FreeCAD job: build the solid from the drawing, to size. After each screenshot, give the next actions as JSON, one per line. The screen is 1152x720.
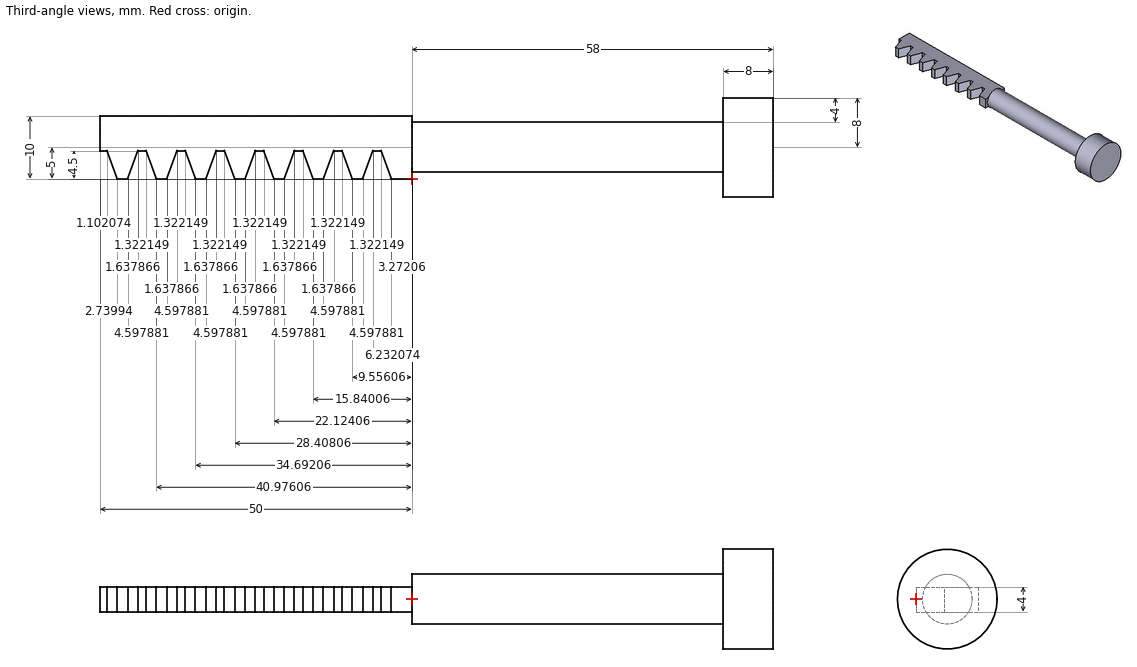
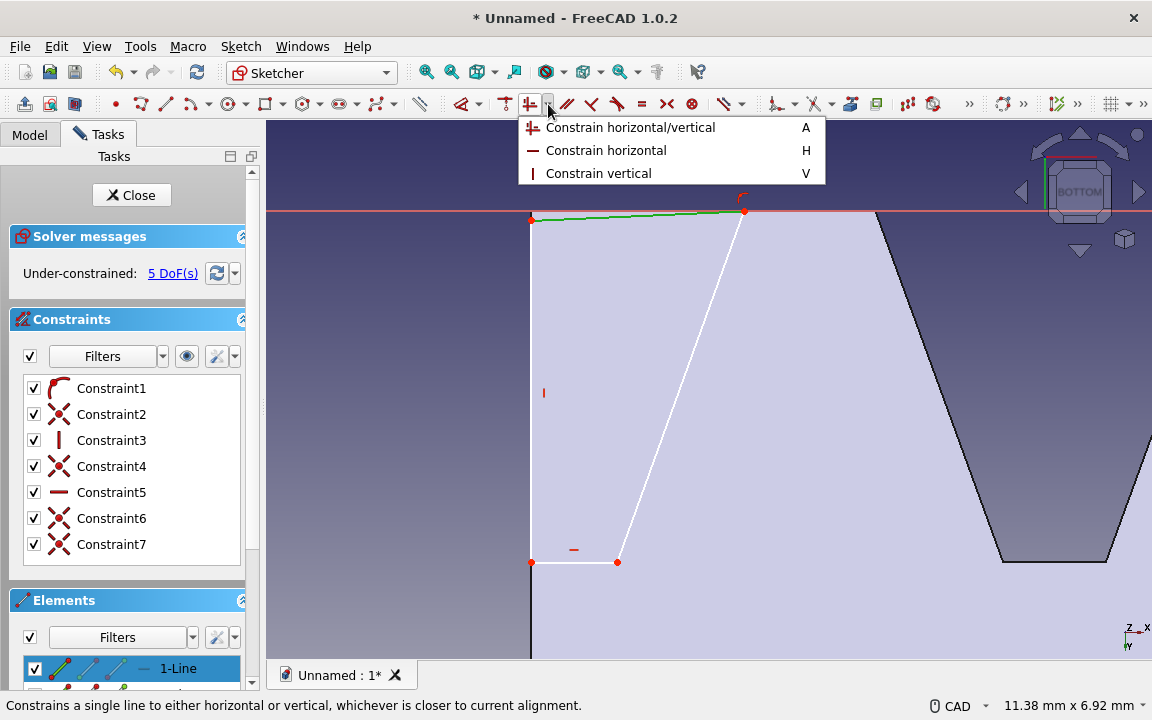
{"action": "left_click", "coordinate": [672, 150]}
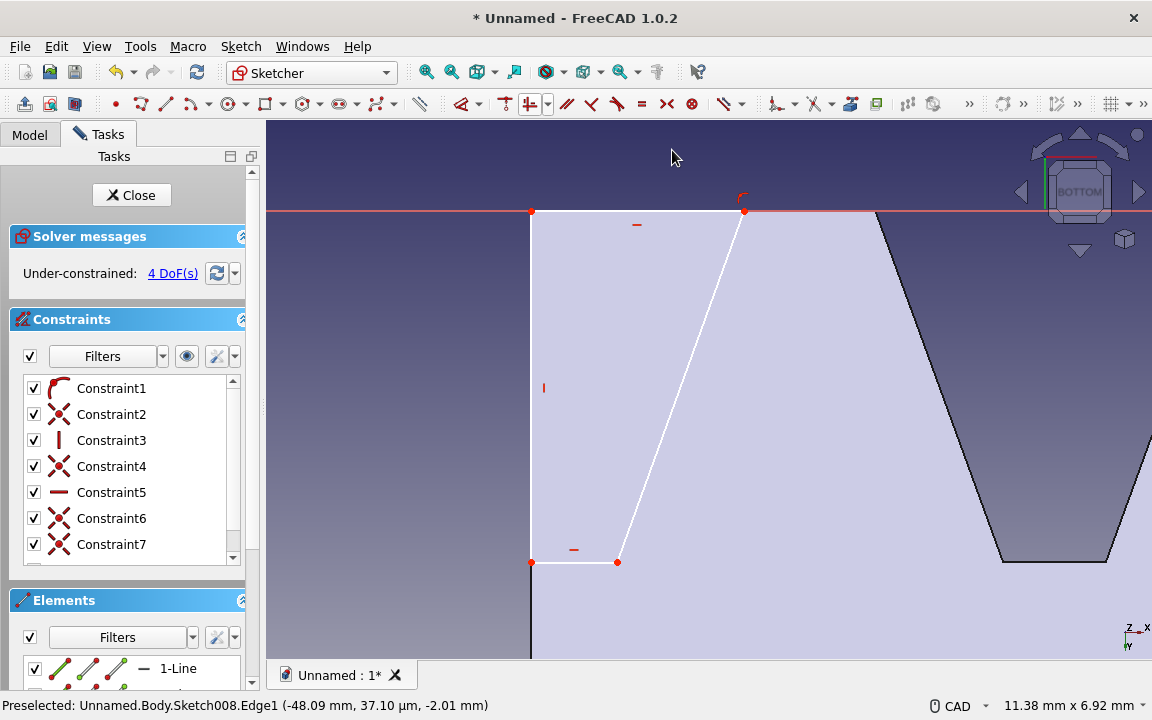
{"action": "left_click", "coordinate": [460, 104]}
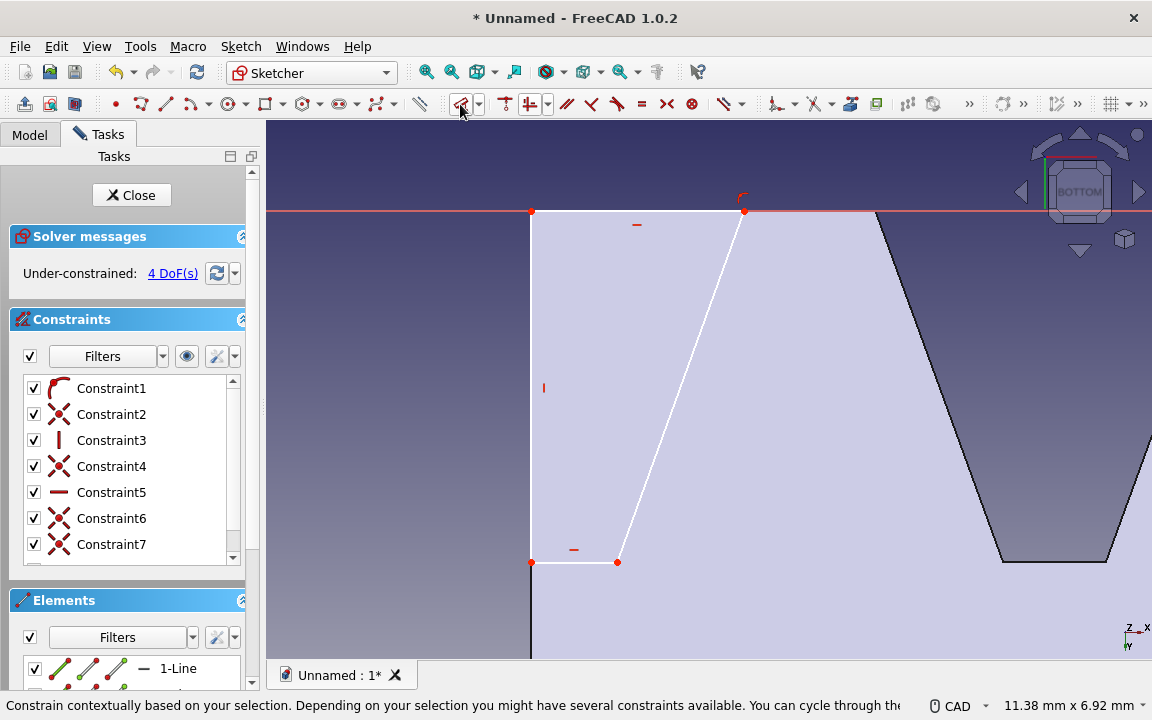
{"action": "left_click", "coordinate": [531, 317]}
{"action": "left_click", "coordinate": [497, 387]}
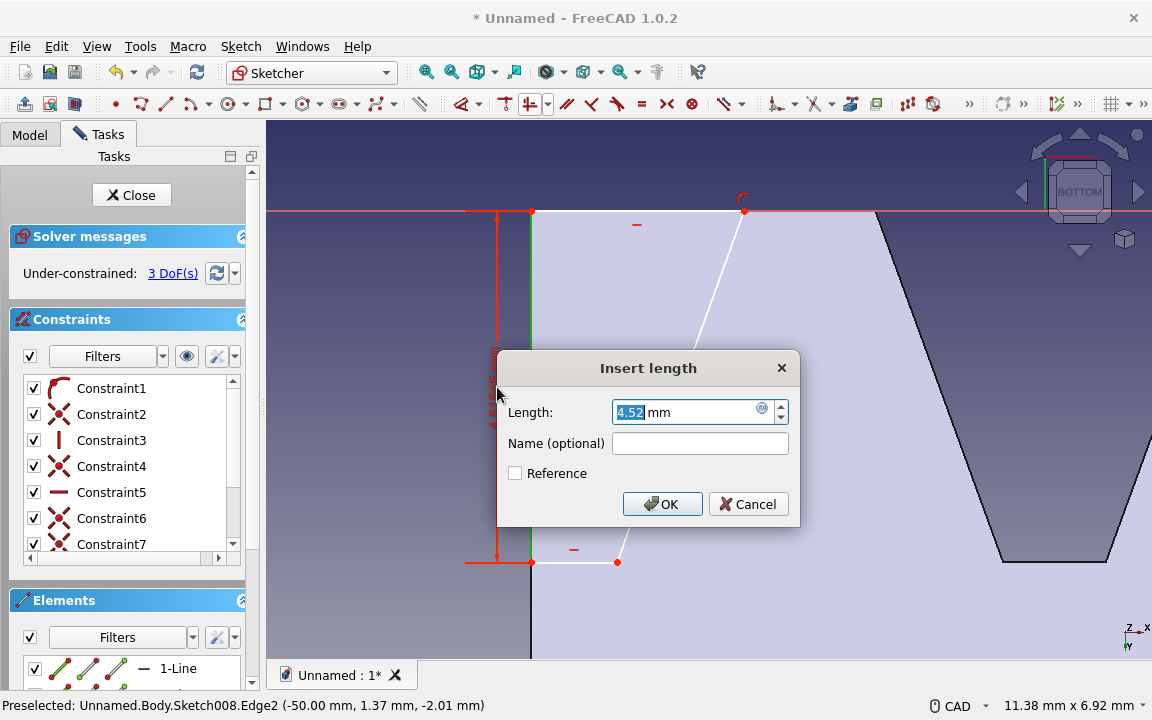
{"action": "type", "text": "4.5"}
{"action": "key", "text": "Return"}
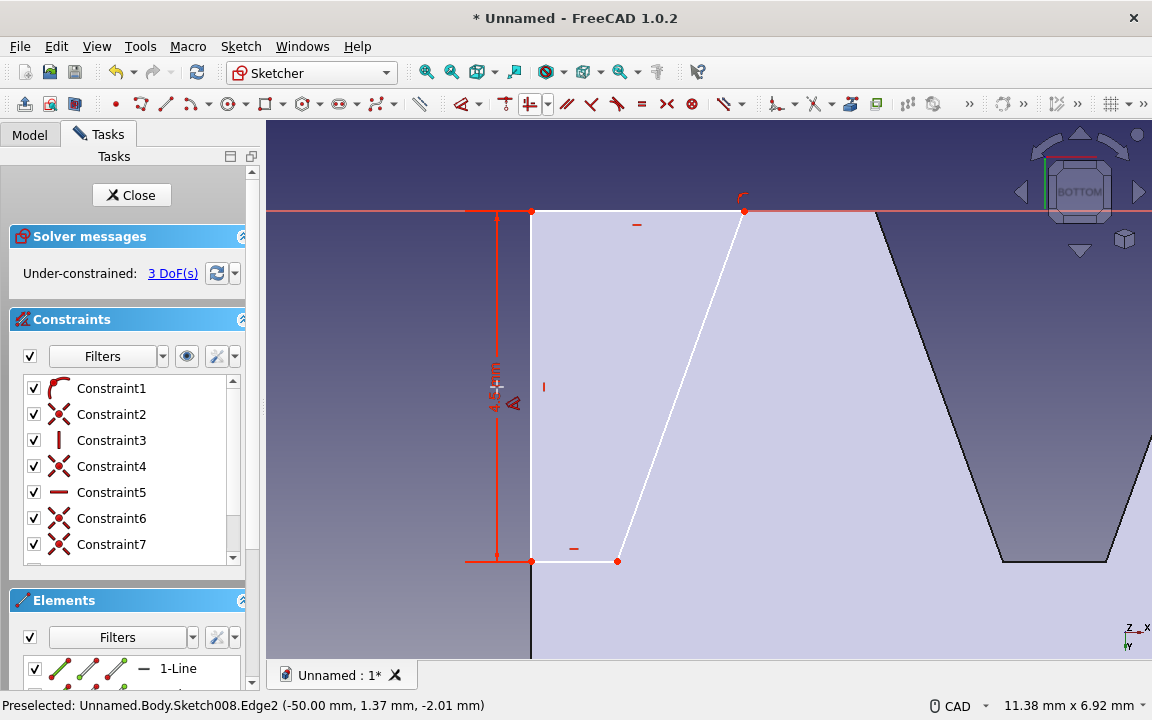
{"action": "left_click", "coordinate": [531, 211]}
{"action": "left_click", "coordinate": [759, 177]}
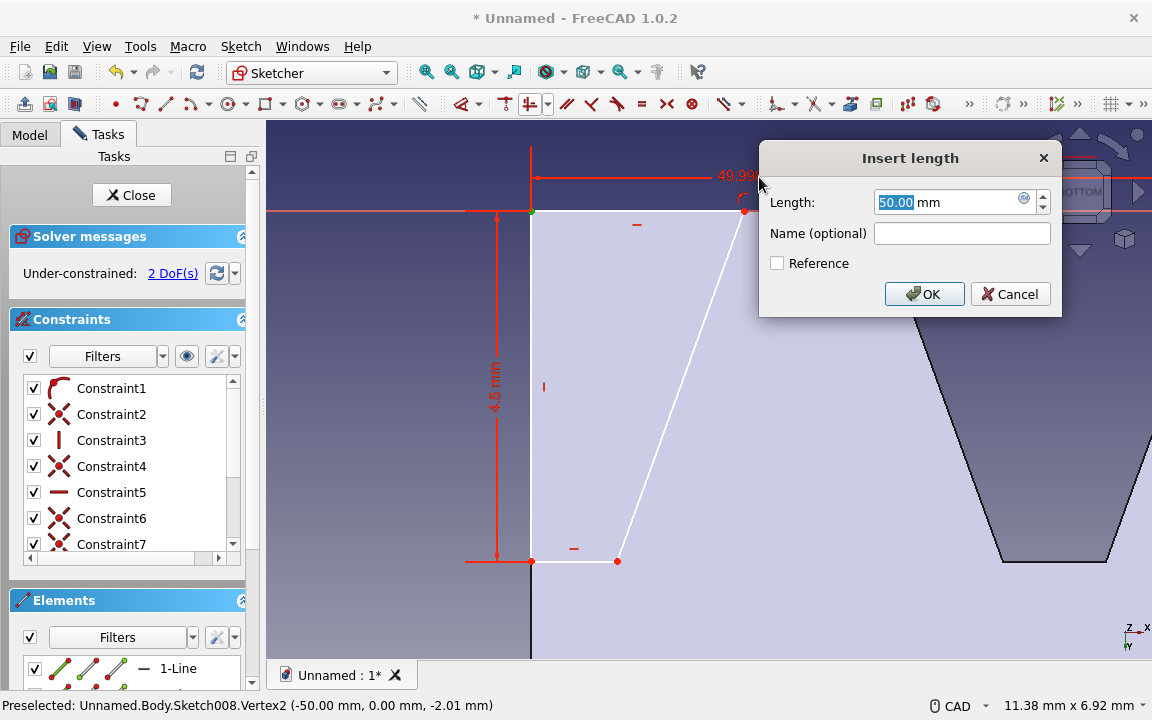
{"action": "type", "text": "50"}
{"action": "key", "text": "Return"}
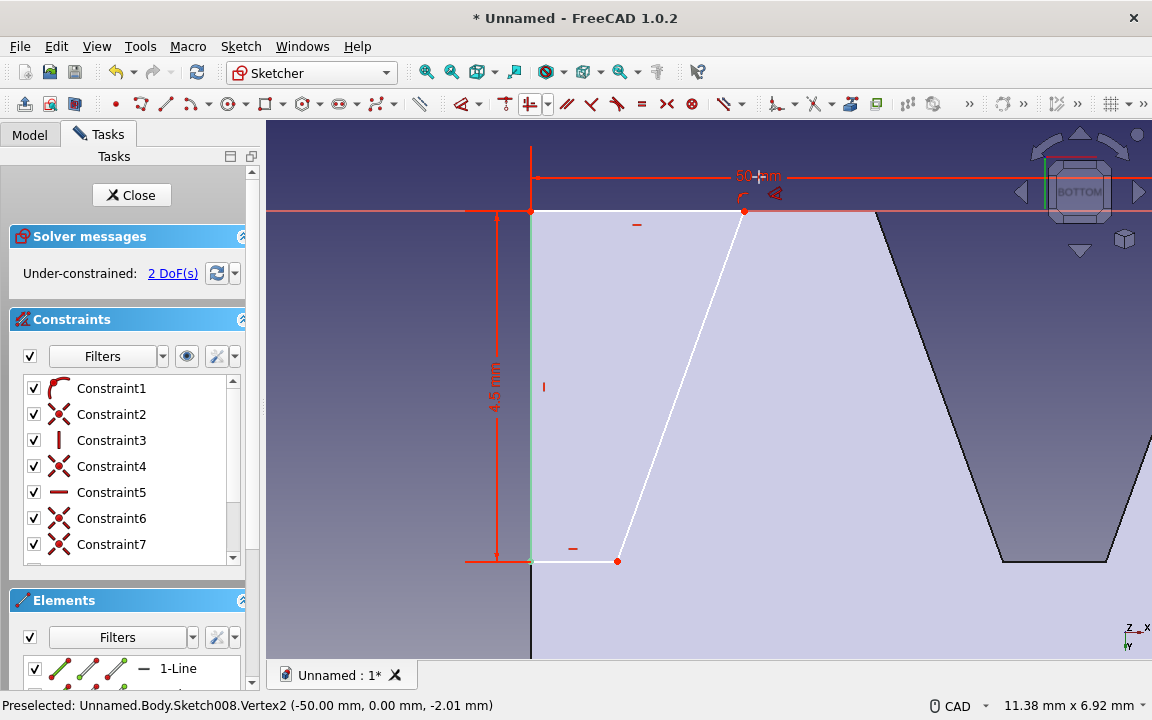
{"action": "left_click", "coordinate": [680, 211]}
{"action": "left_click", "coordinate": [637, 177]}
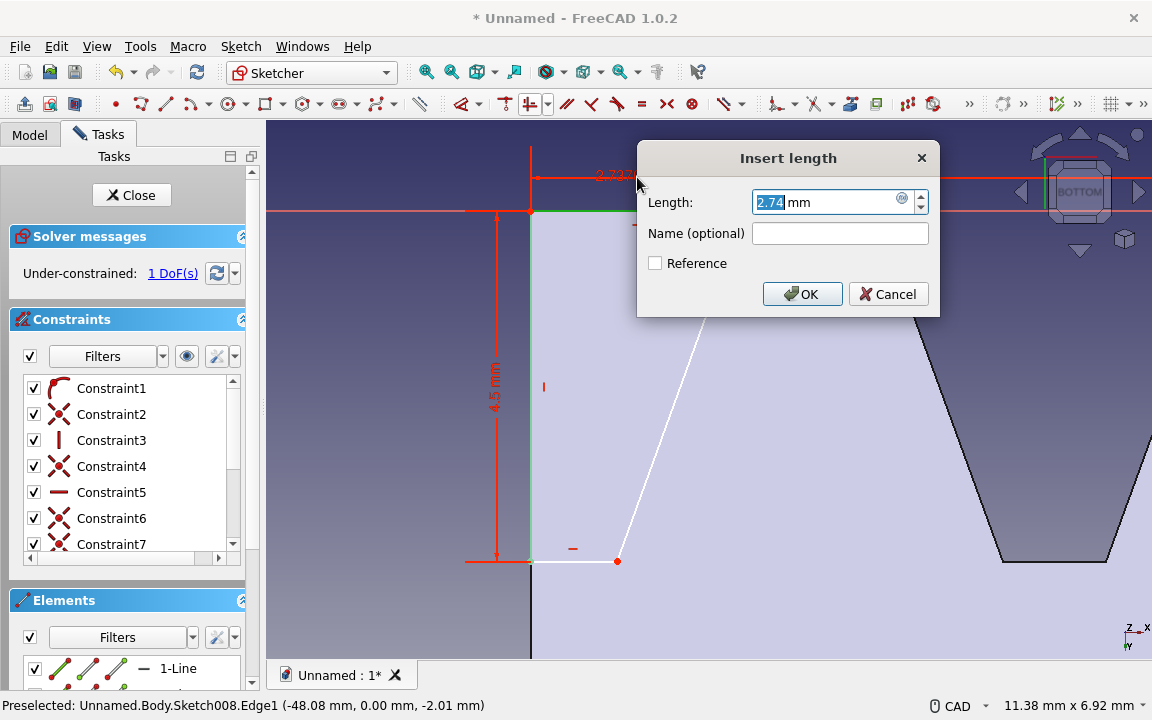
{"action": "type", "text": "2.73994"}
{"action": "key", "text": "Return"}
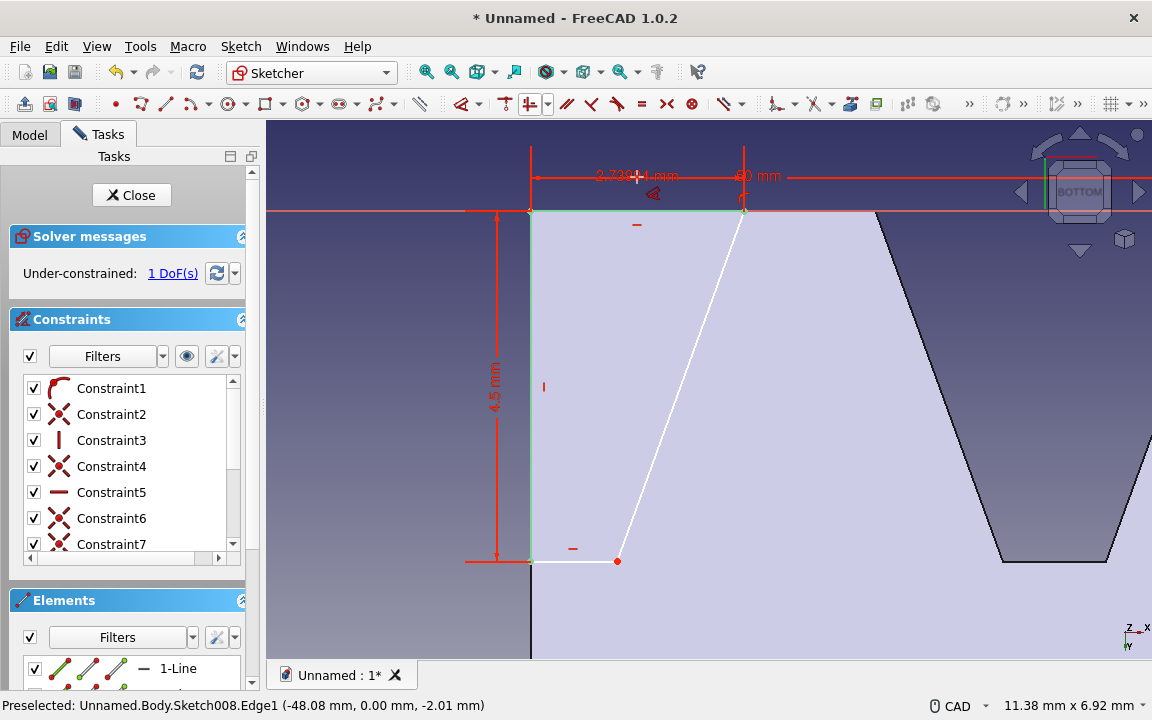
{"action": "left_click", "coordinate": [557, 562]}
{"action": "left_click", "coordinate": [574, 596]}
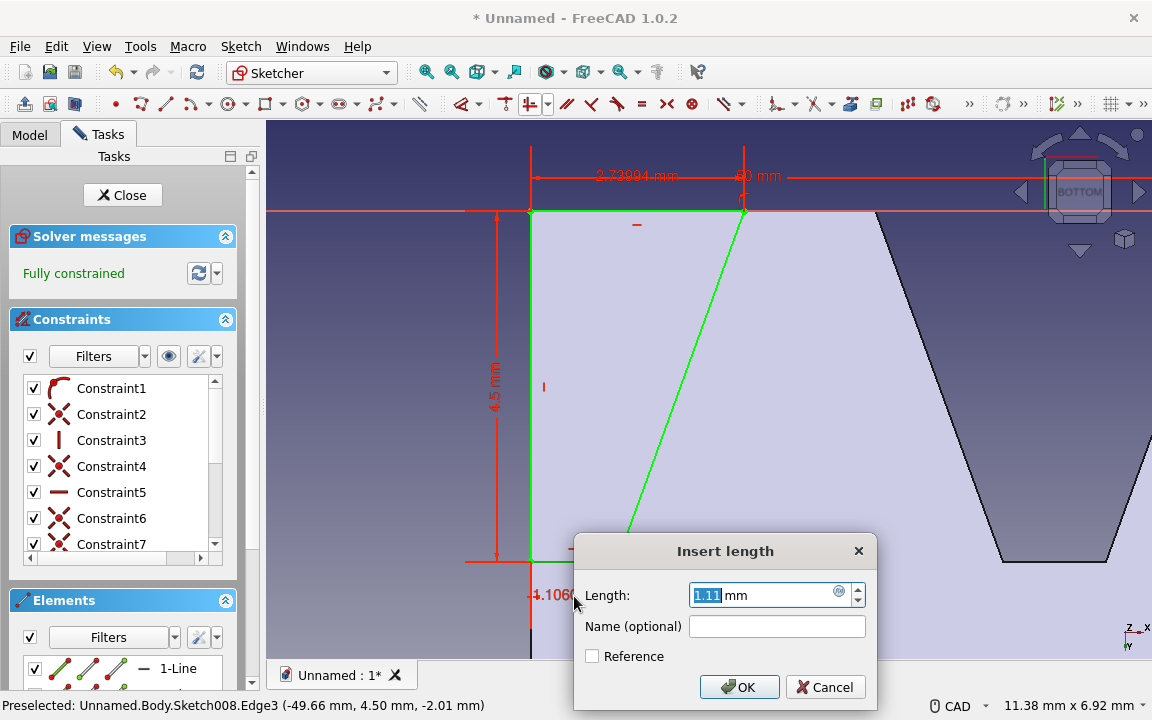
{"action": "type", "text": "1.102074"}
{"action": "key", "text": "Return"}
{"action": "key", "text": "Escape"}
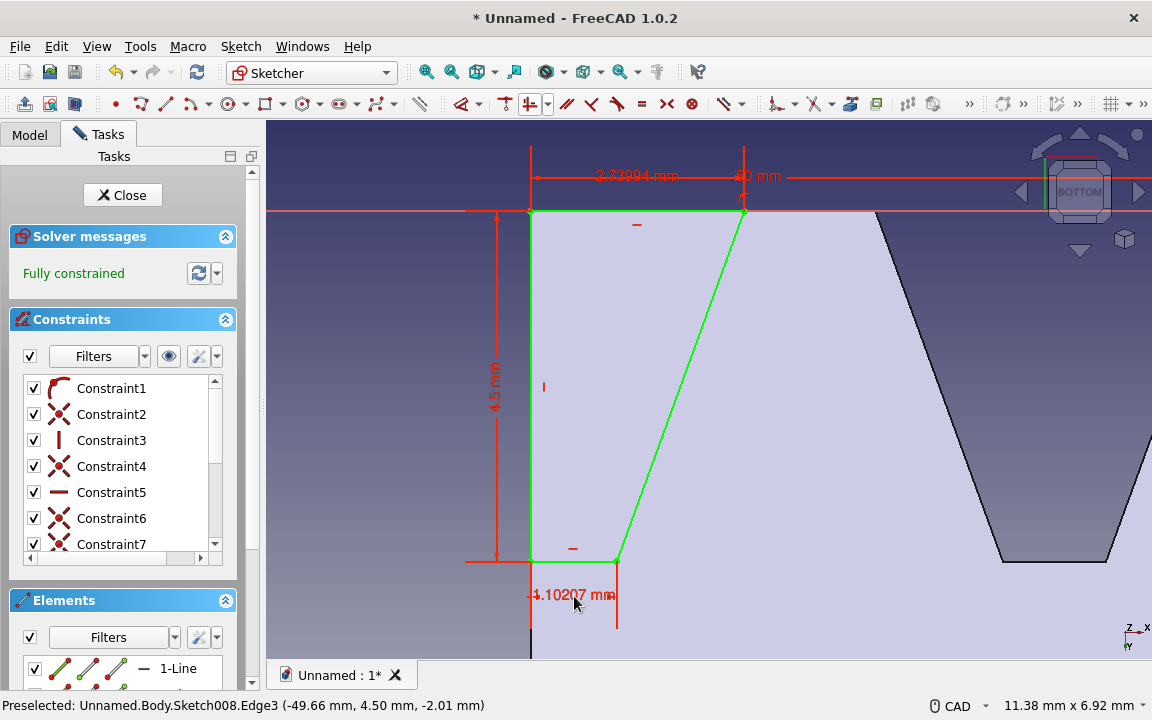
{"action": "left_click", "coordinate": [123, 195]}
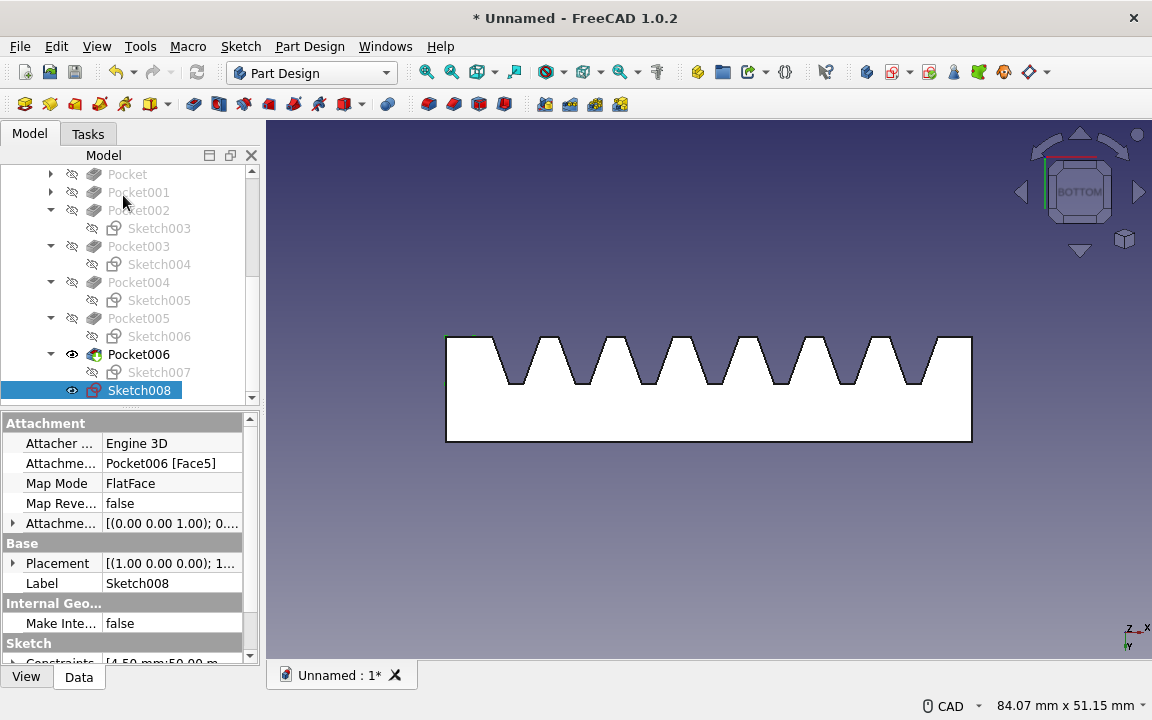
{"action": "left_click", "coordinate": [194, 104]}